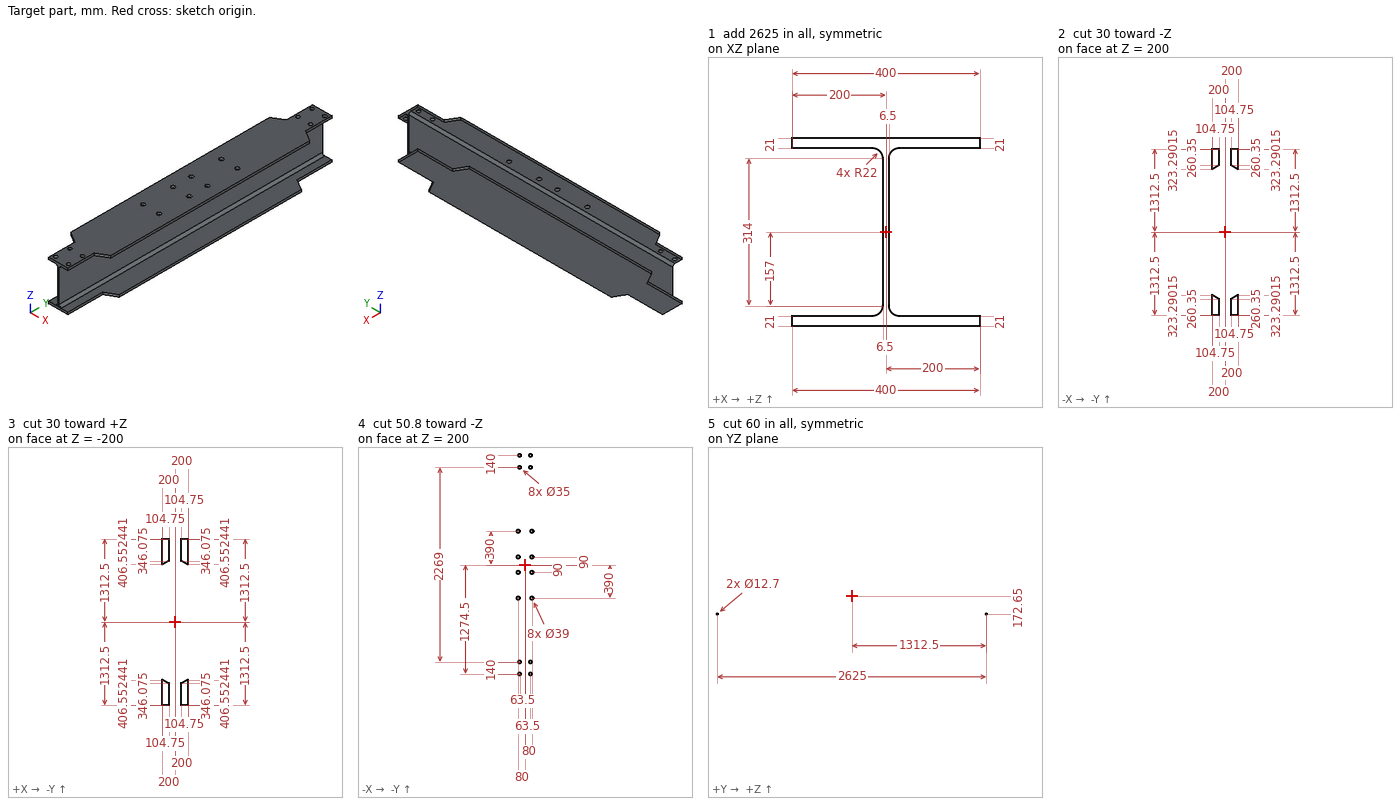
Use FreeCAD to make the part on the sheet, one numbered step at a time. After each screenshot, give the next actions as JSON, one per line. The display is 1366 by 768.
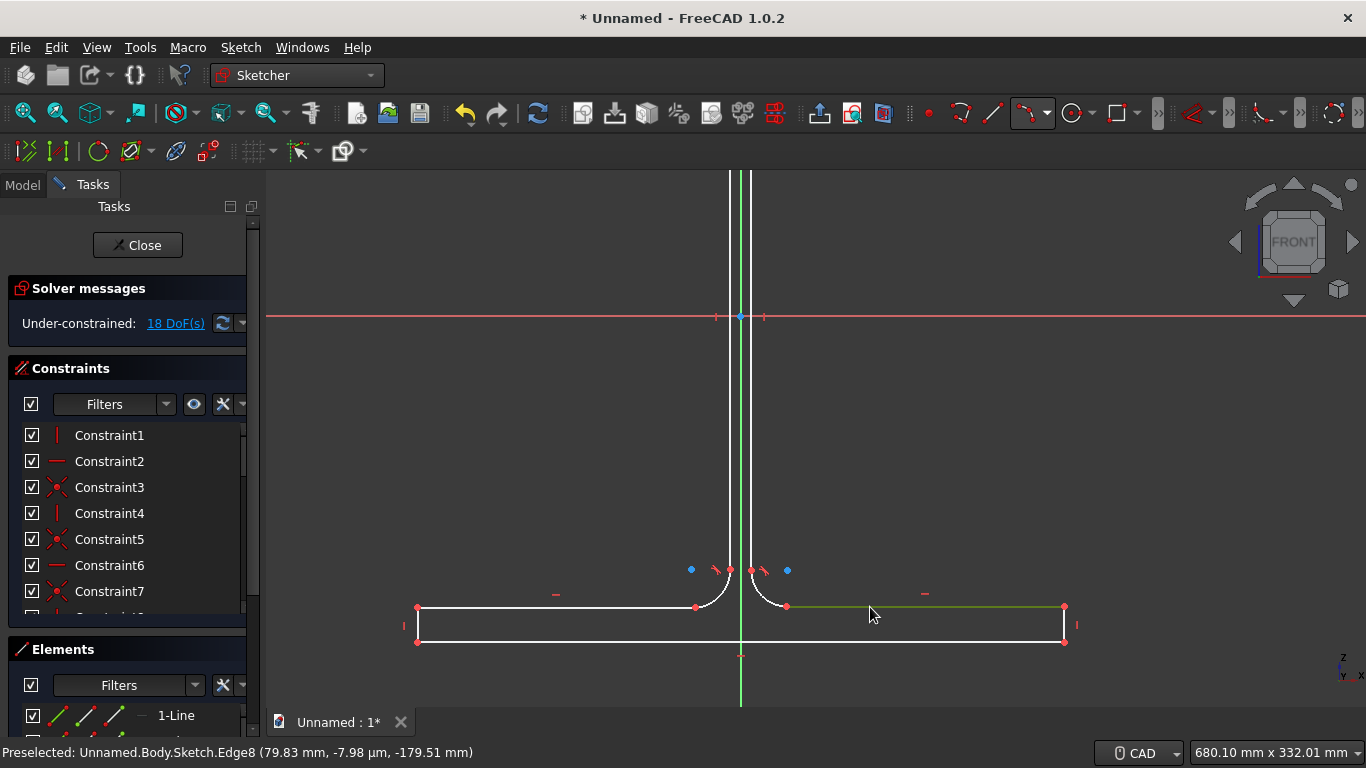
{"action": "left_click", "coordinate": [755, 587]}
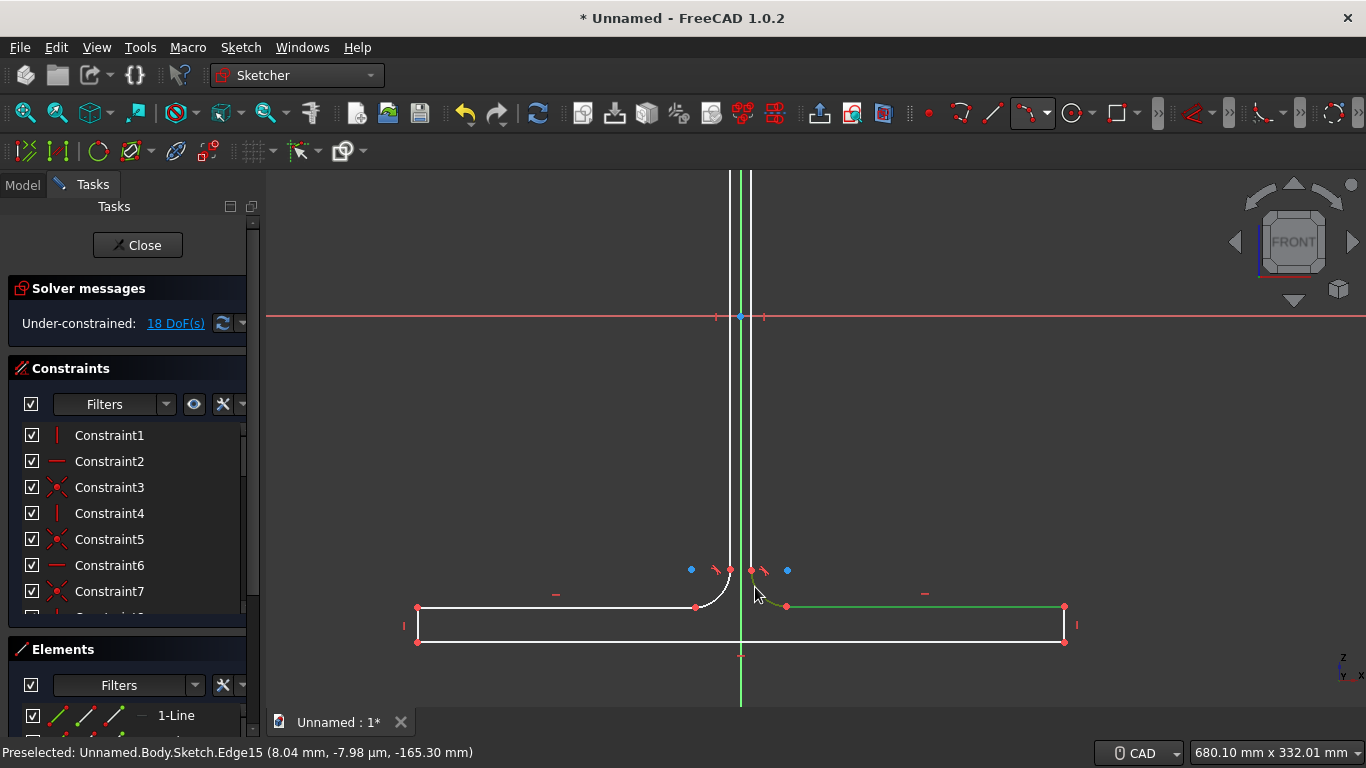
{"action": "key", "text": "t"}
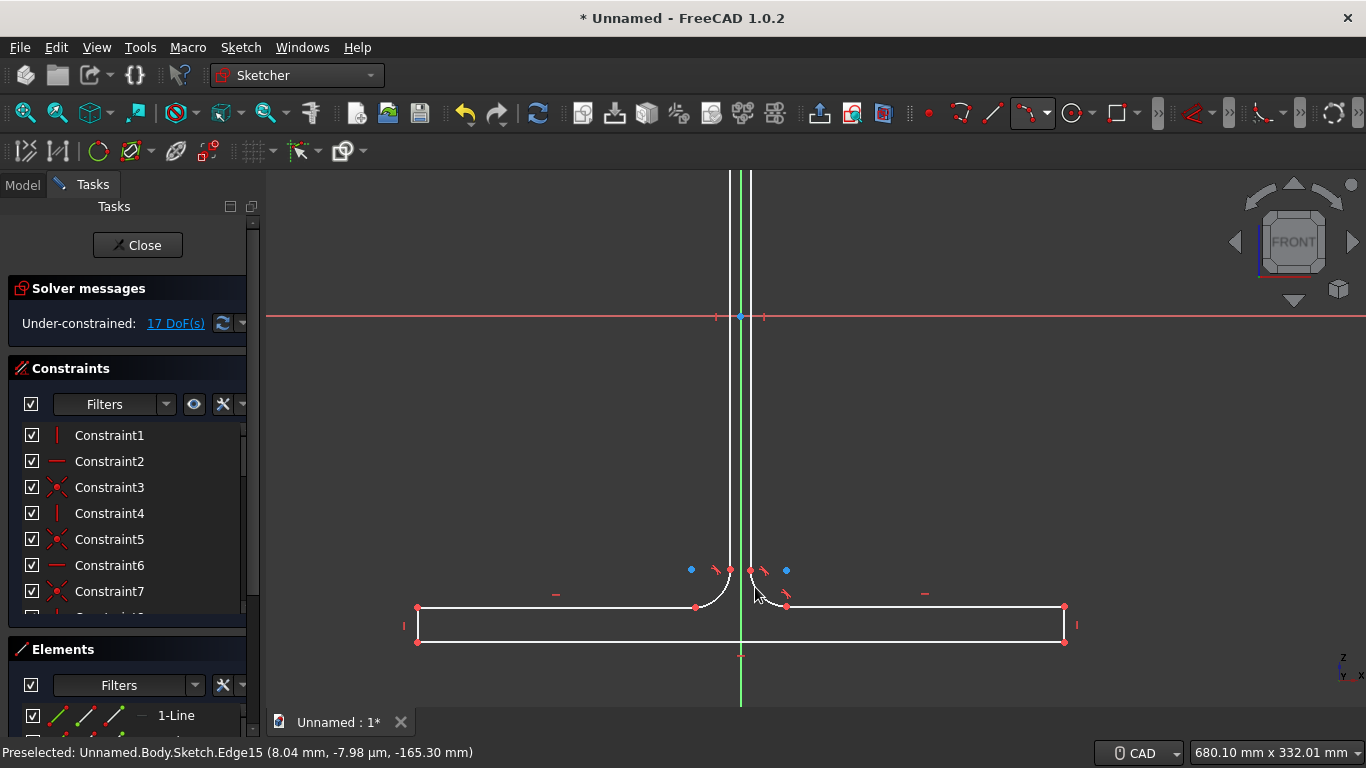
{"action": "left_click", "coordinate": [501, 608]}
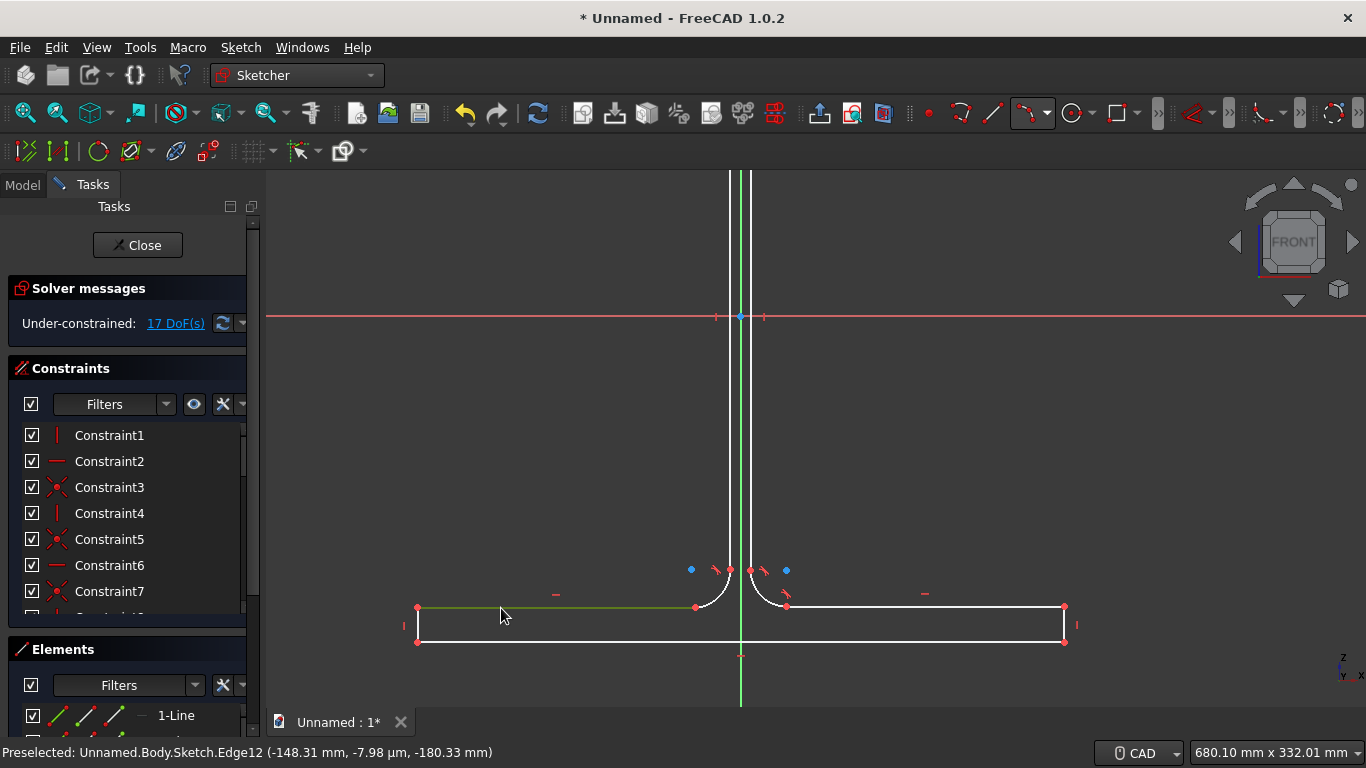
{"action": "left_click", "coordinate": [712, 603]}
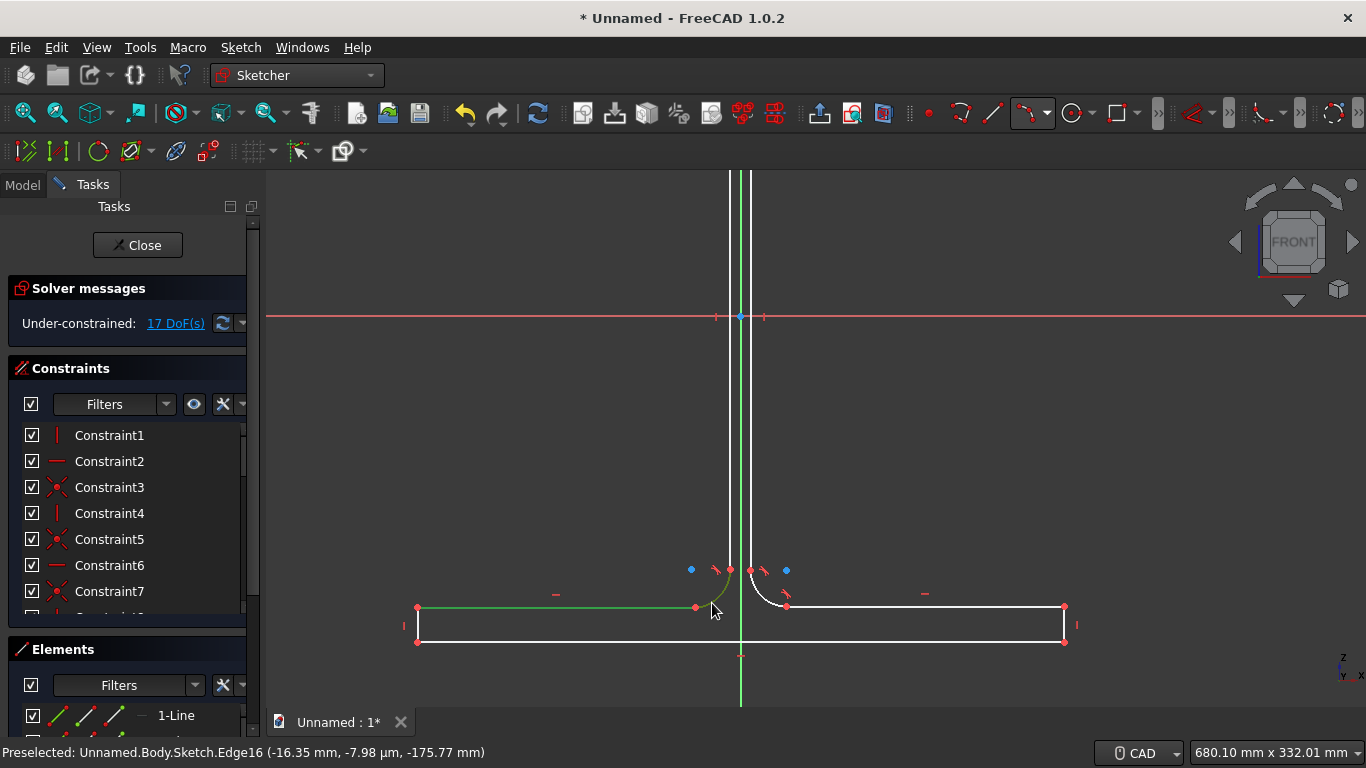
{"action": "key", "text": "t"}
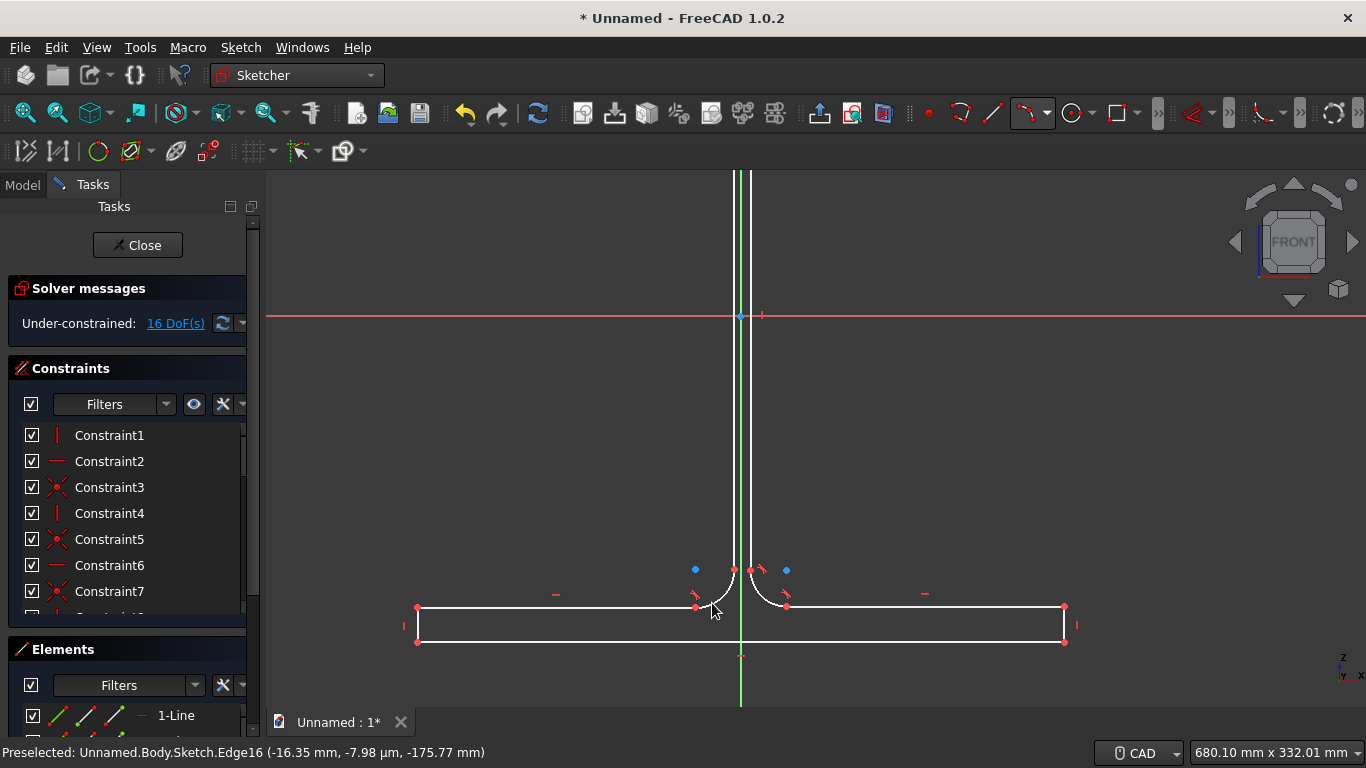
{"action": "scroll", "coordinate": [756, 587], "scroll_direction": "down", "scroll_amount": 3}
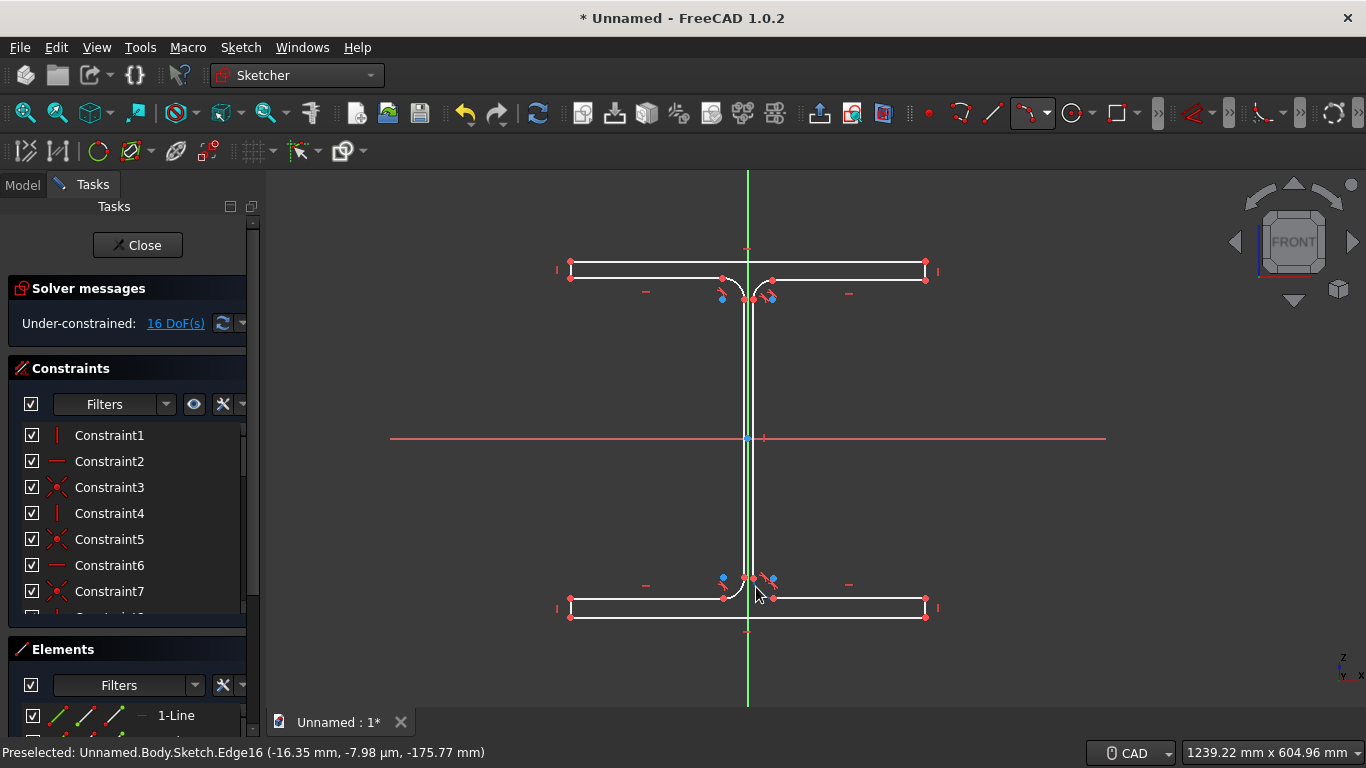
{"action": "scroll", "coordinate": [742, 290], "scroll_direction": "up", "scroll_amount": 5}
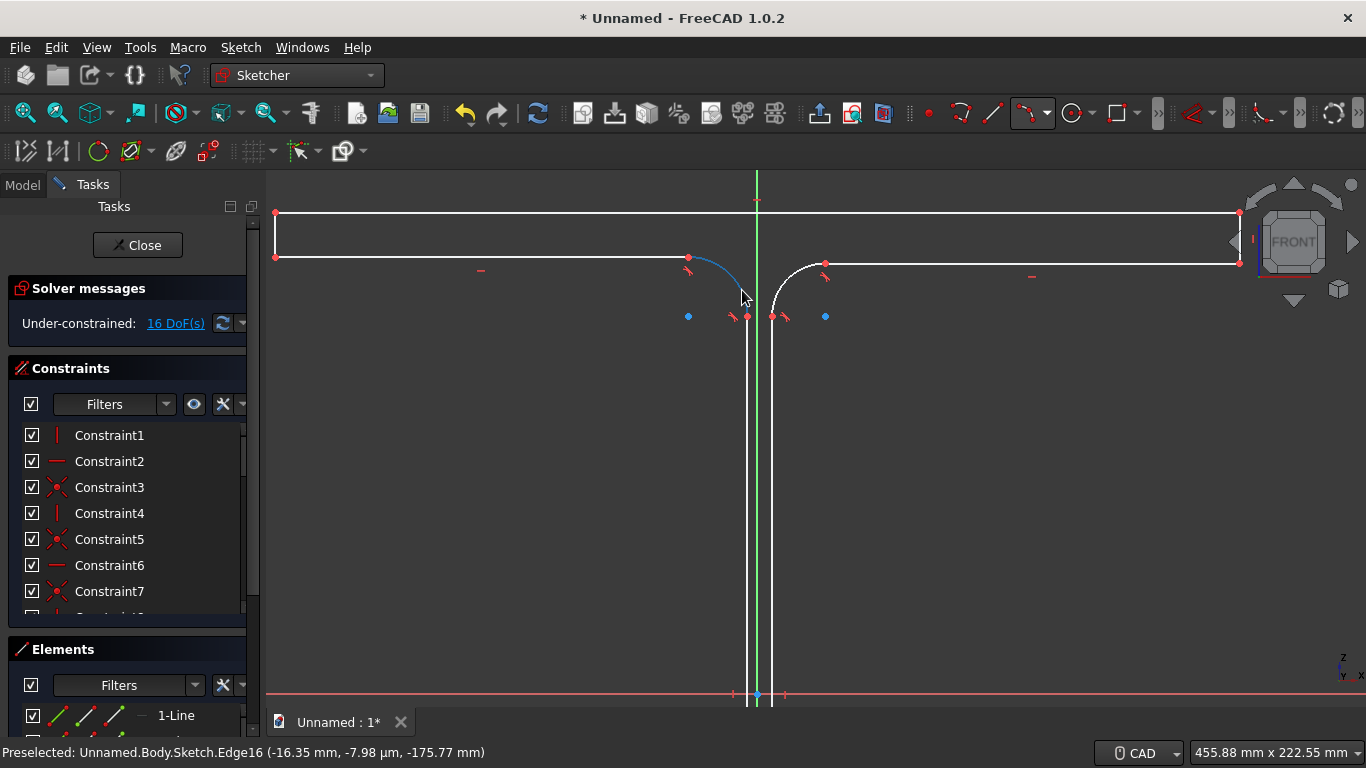
{"action": "left_click", "coordinate": [741, 289]}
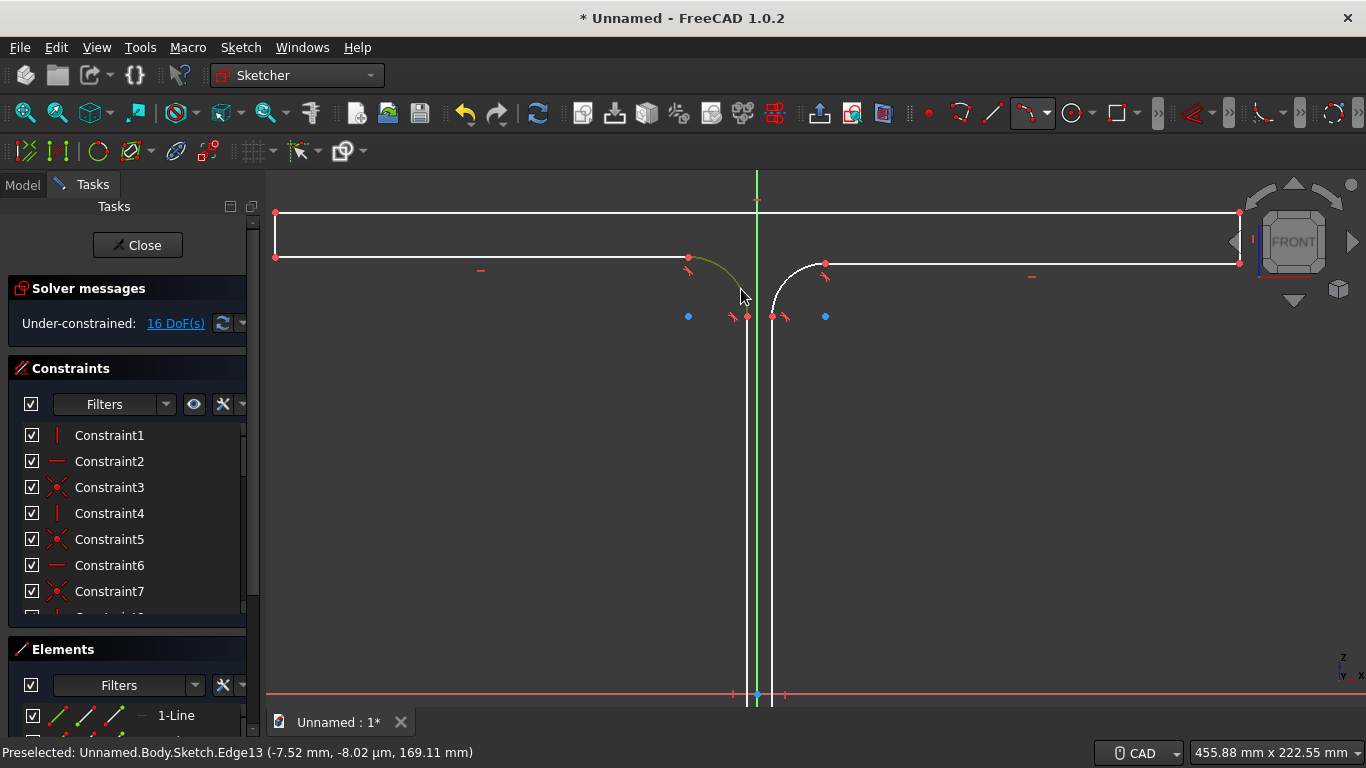
{"action": "left_click", "coordinate": [801, 269]}